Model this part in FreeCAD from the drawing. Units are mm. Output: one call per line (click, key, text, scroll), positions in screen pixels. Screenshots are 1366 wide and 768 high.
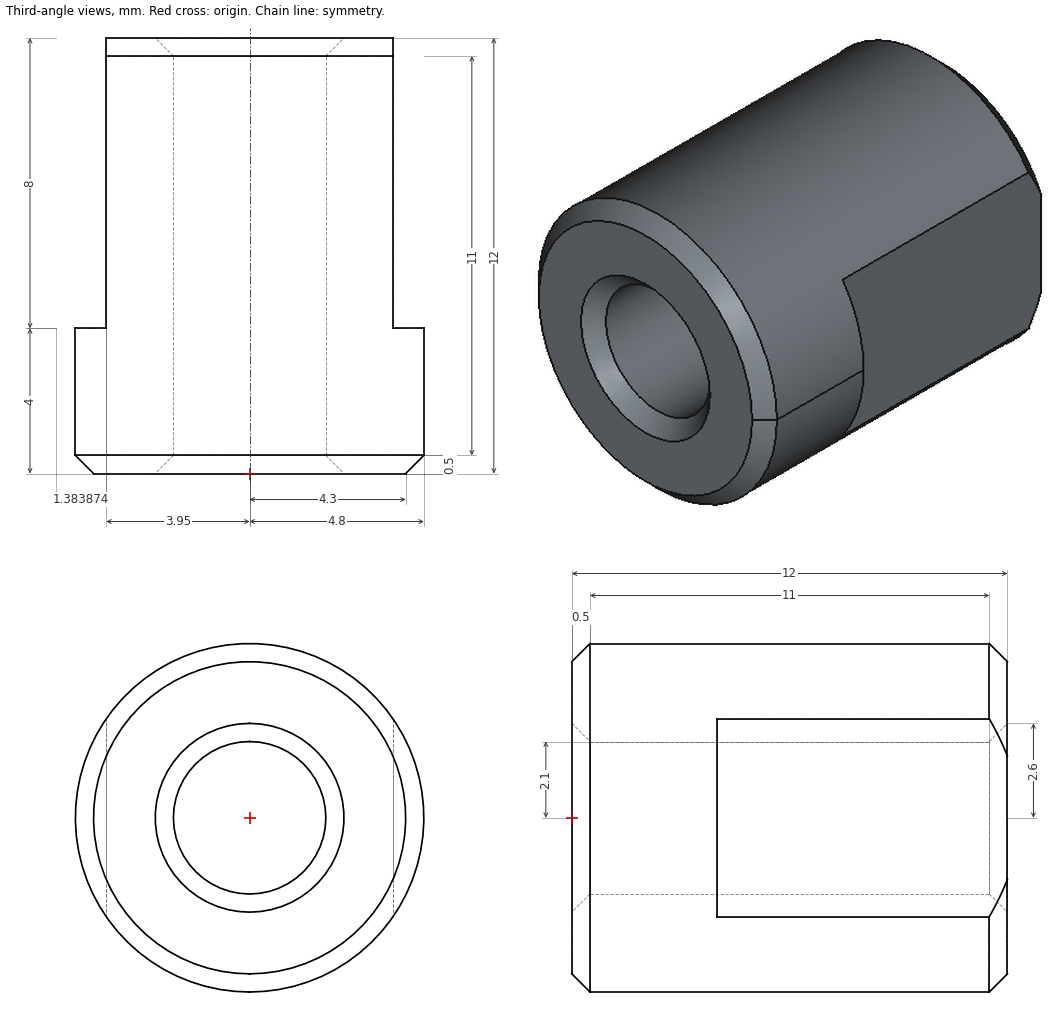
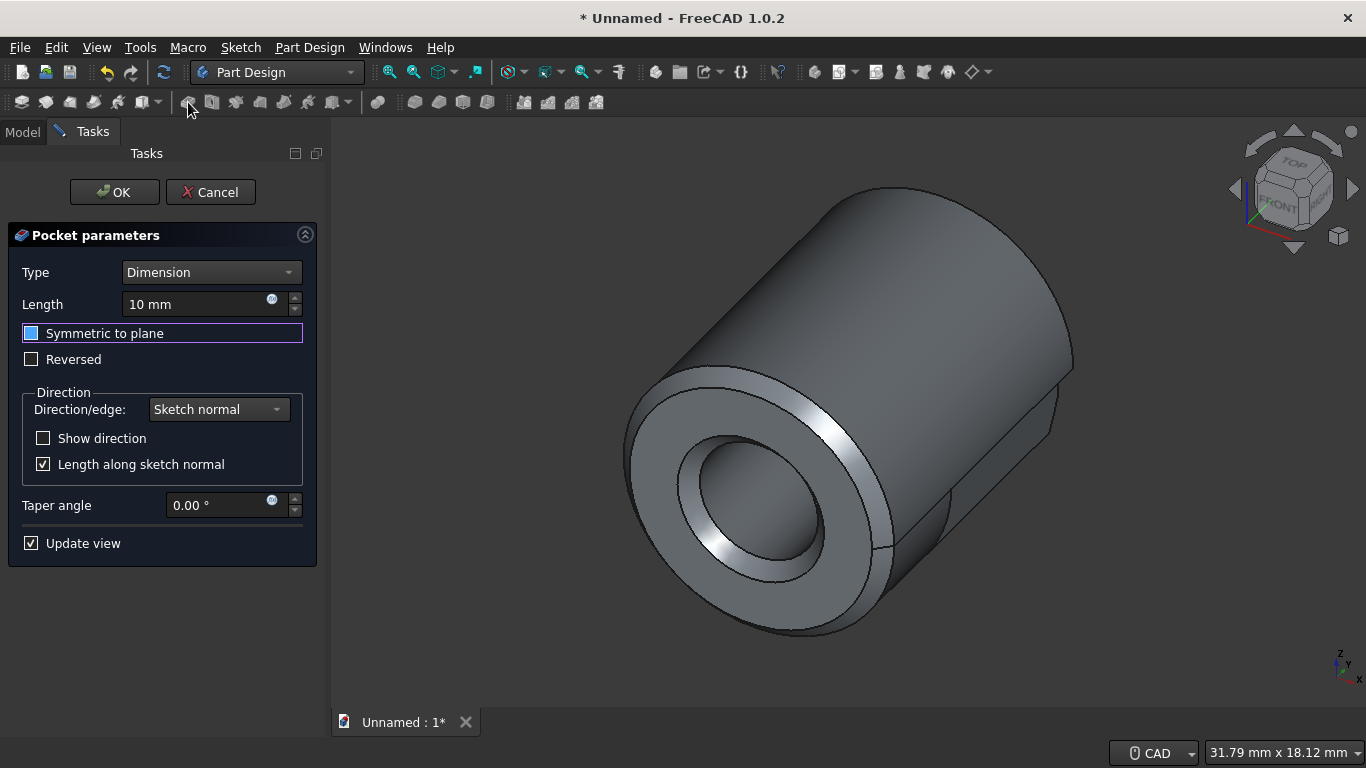
click(30, 333)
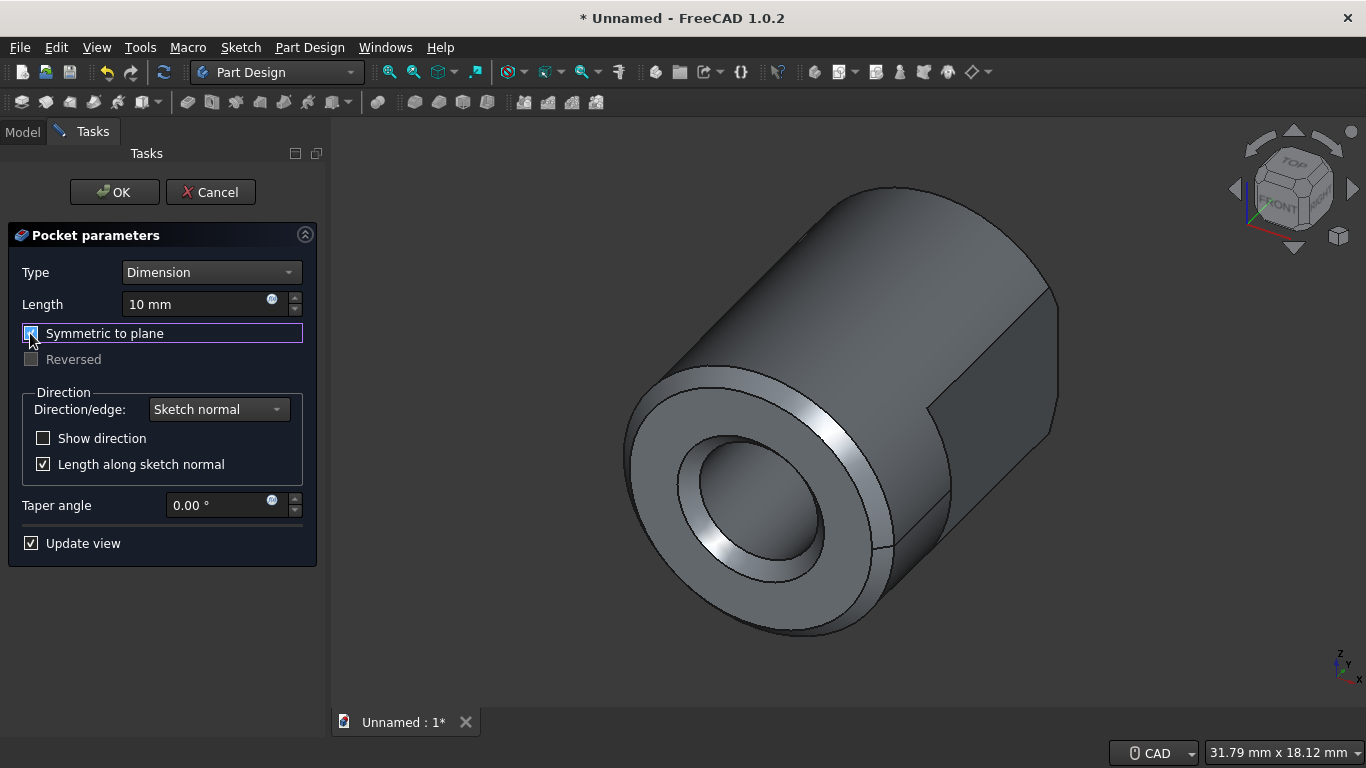
click(115, 192)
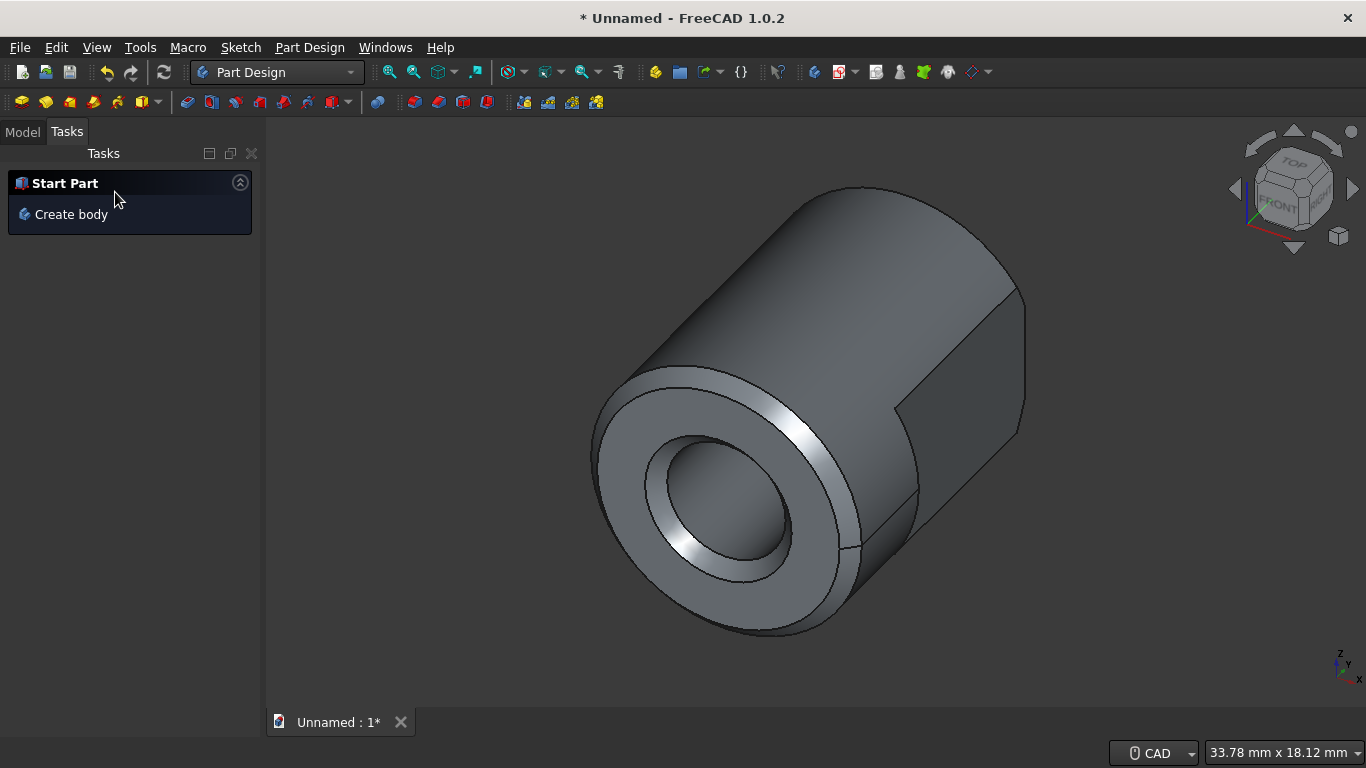
key(0)